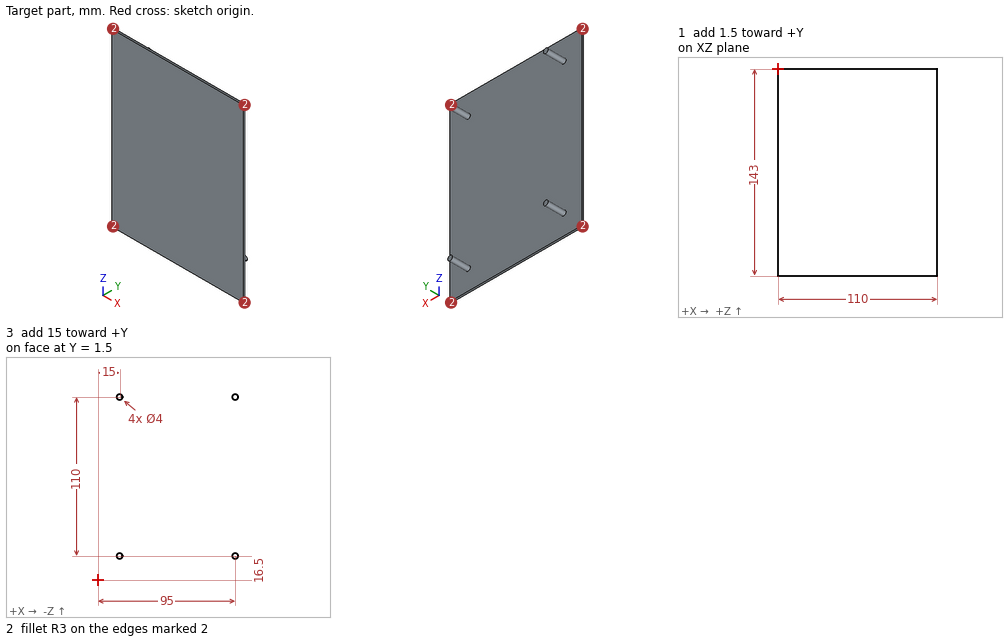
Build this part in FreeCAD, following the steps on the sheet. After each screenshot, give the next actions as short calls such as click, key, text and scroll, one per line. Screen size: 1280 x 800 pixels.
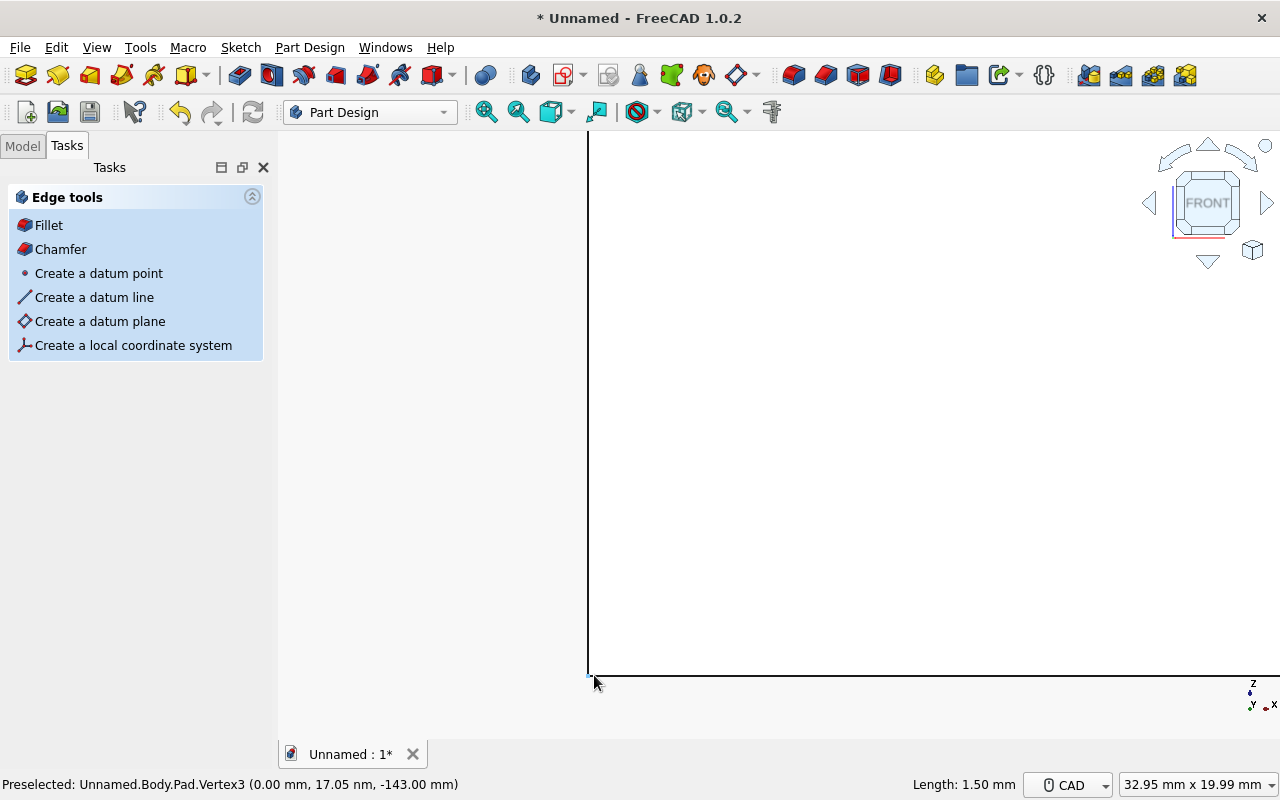
click(488, 112)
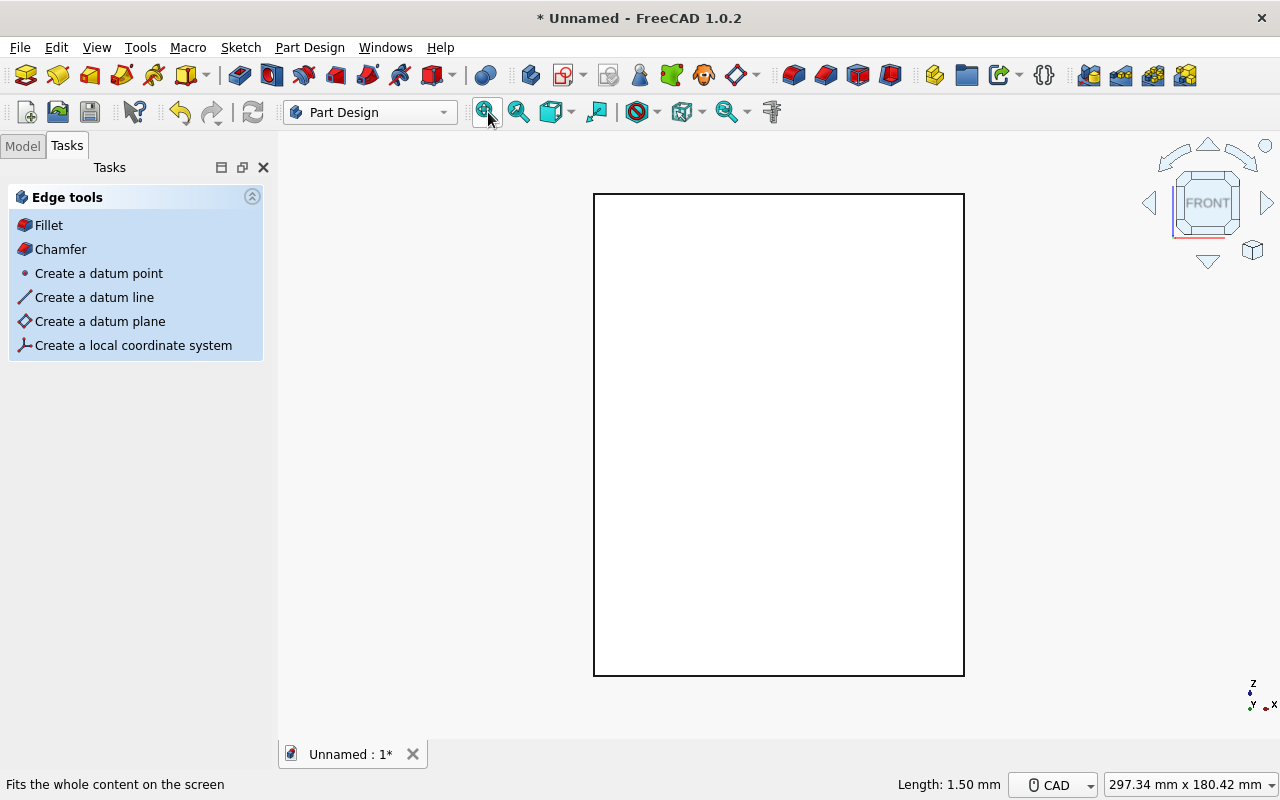
key(3)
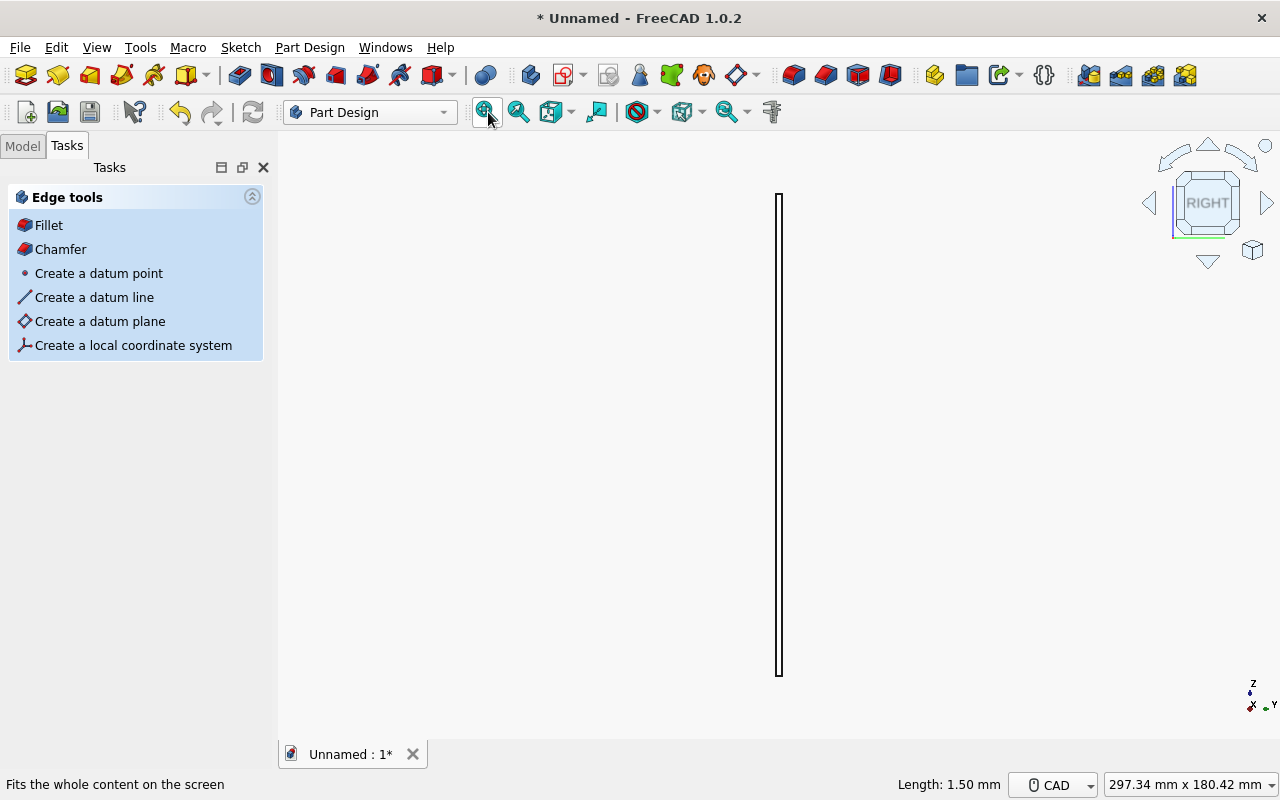
scroll(779, 675, up, 11)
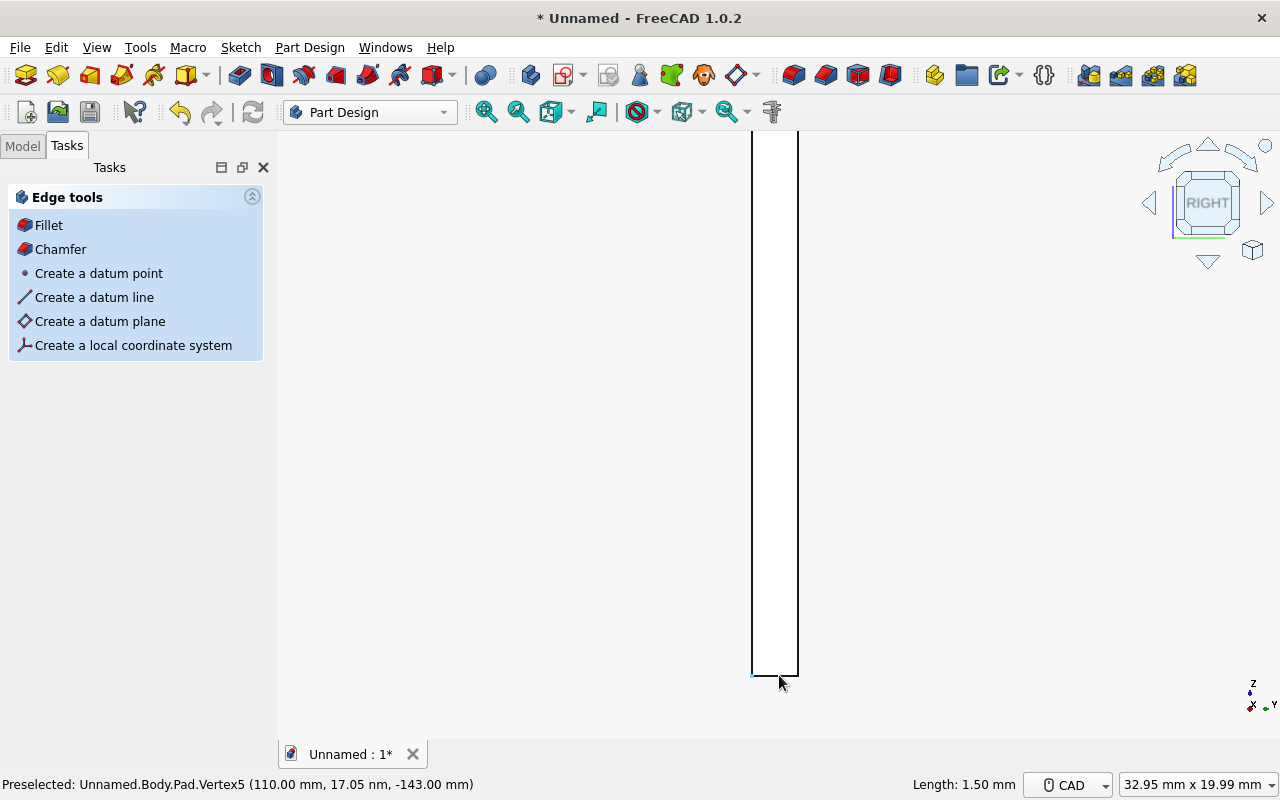
click(775, 675, ctrl)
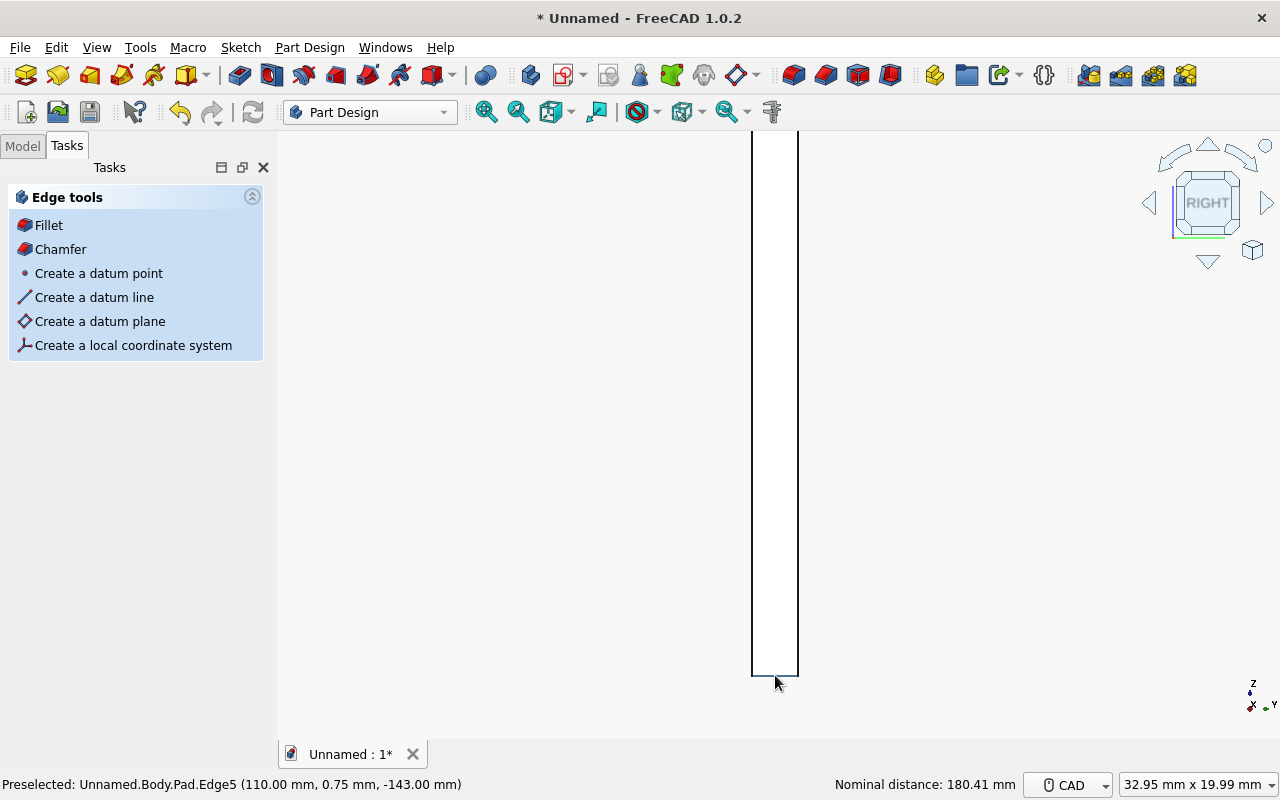
click(488, 112)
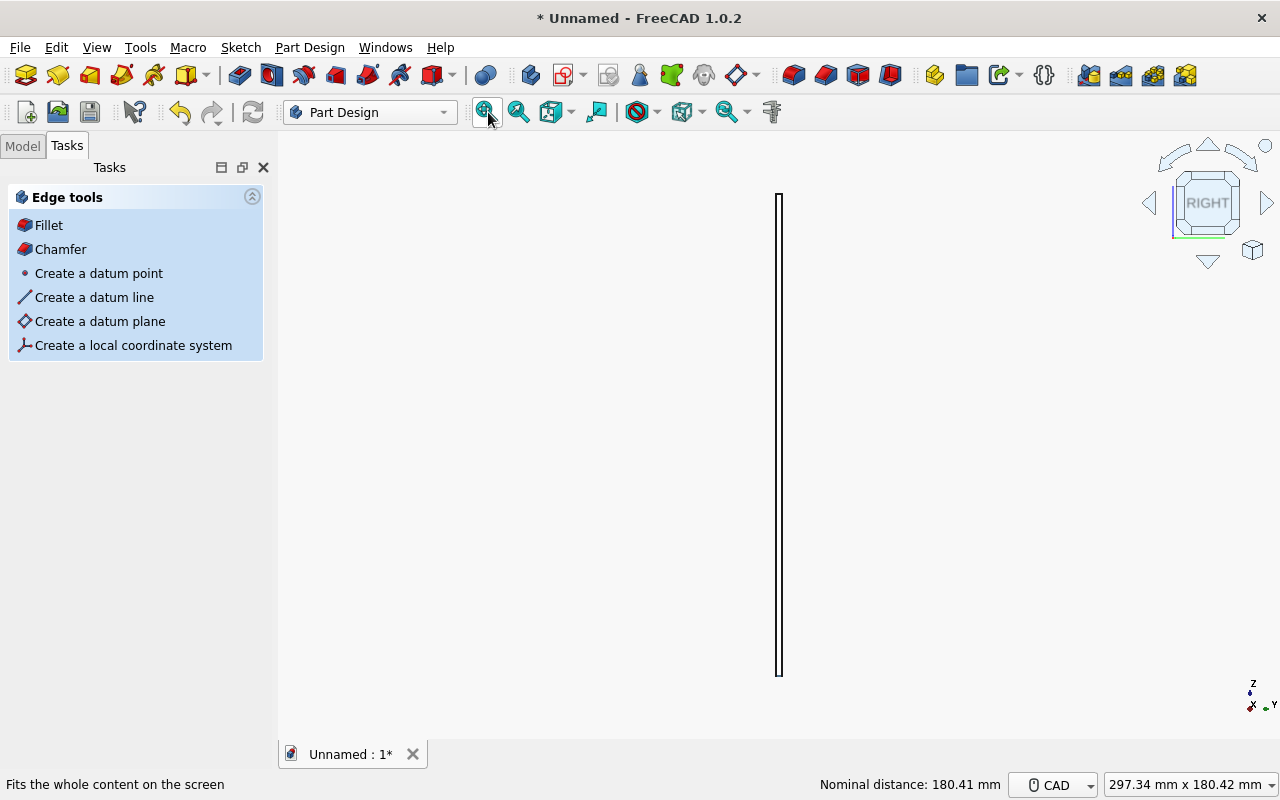
key(5)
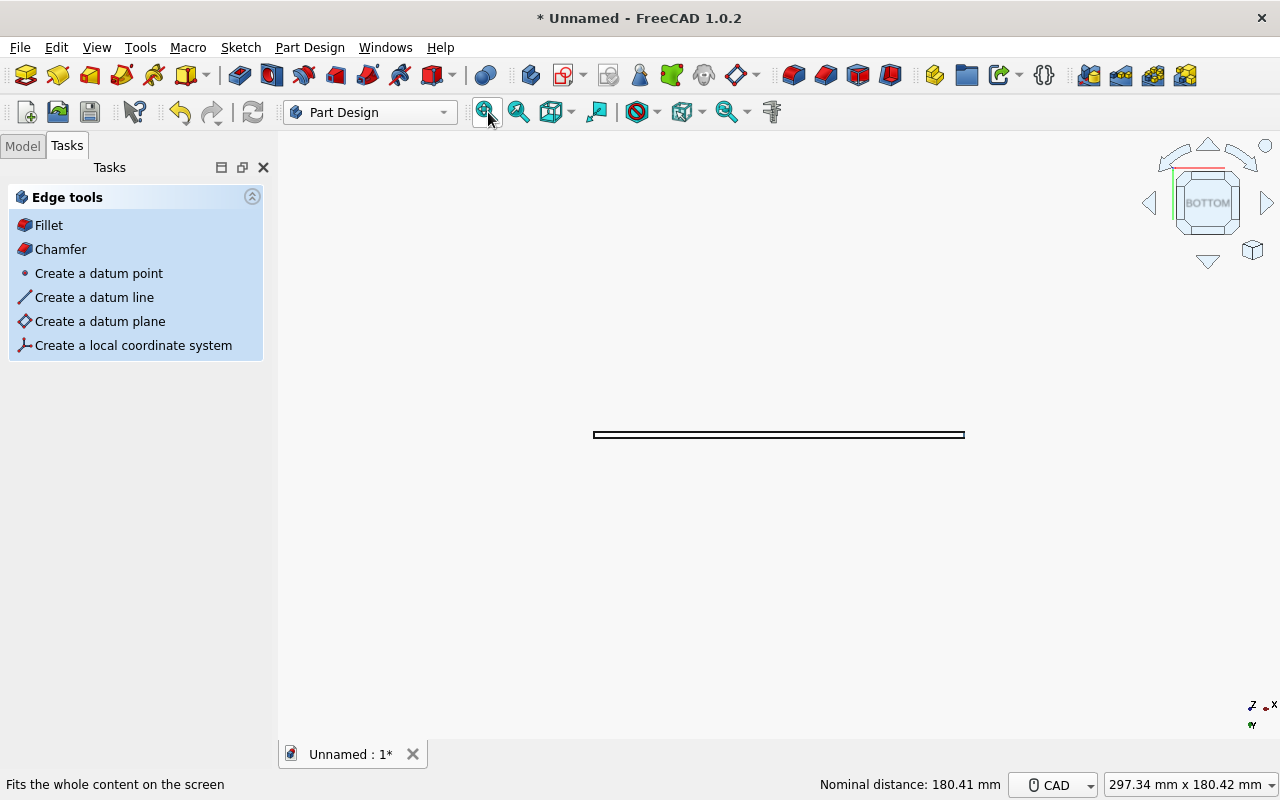
click(488, 112)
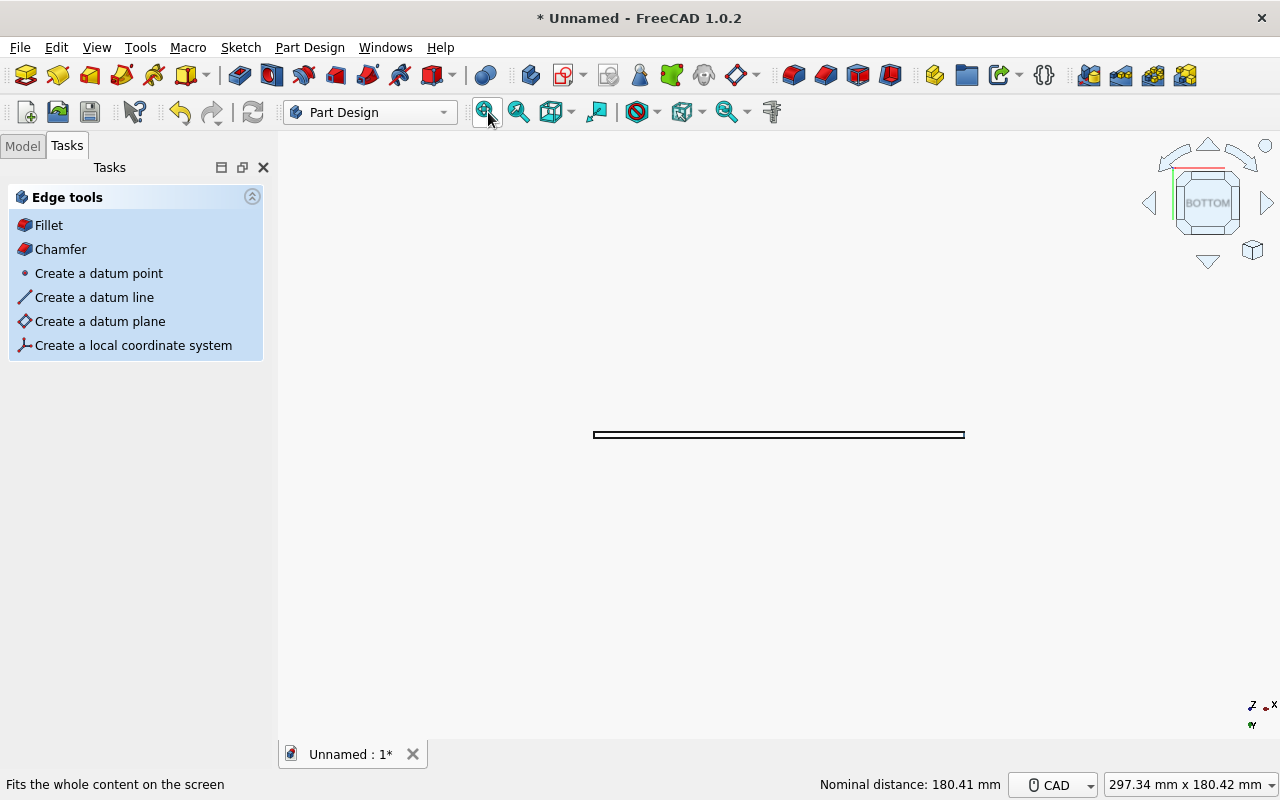
scroll(594, 434, up, 11)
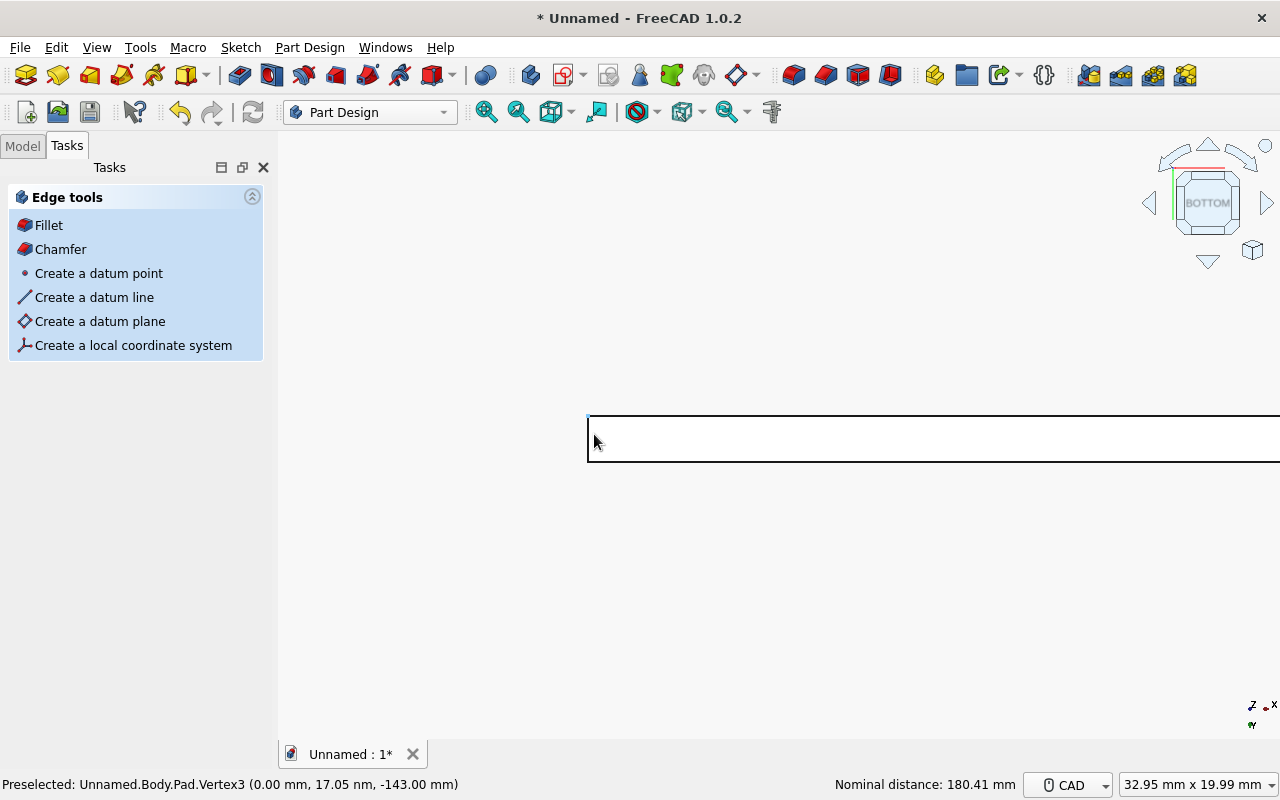
click(588, 438, ctrl)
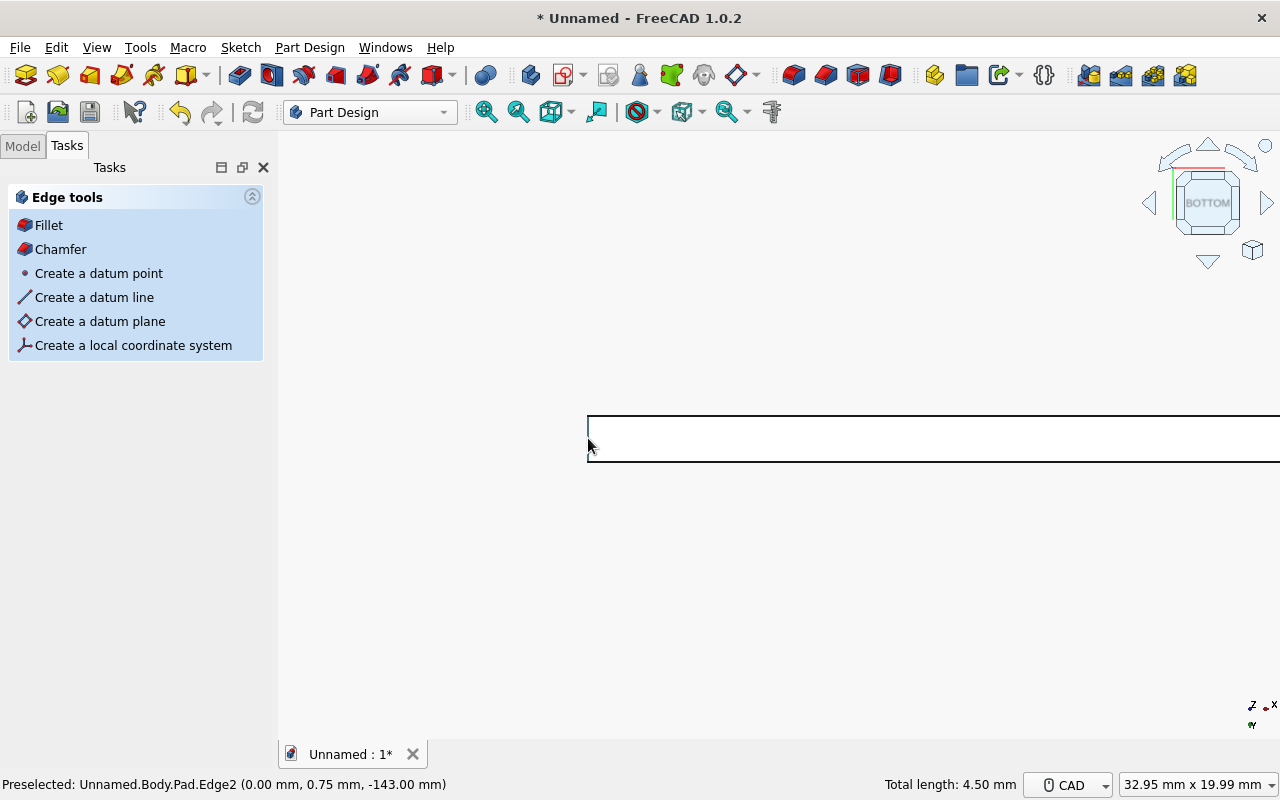
click(488, 112)